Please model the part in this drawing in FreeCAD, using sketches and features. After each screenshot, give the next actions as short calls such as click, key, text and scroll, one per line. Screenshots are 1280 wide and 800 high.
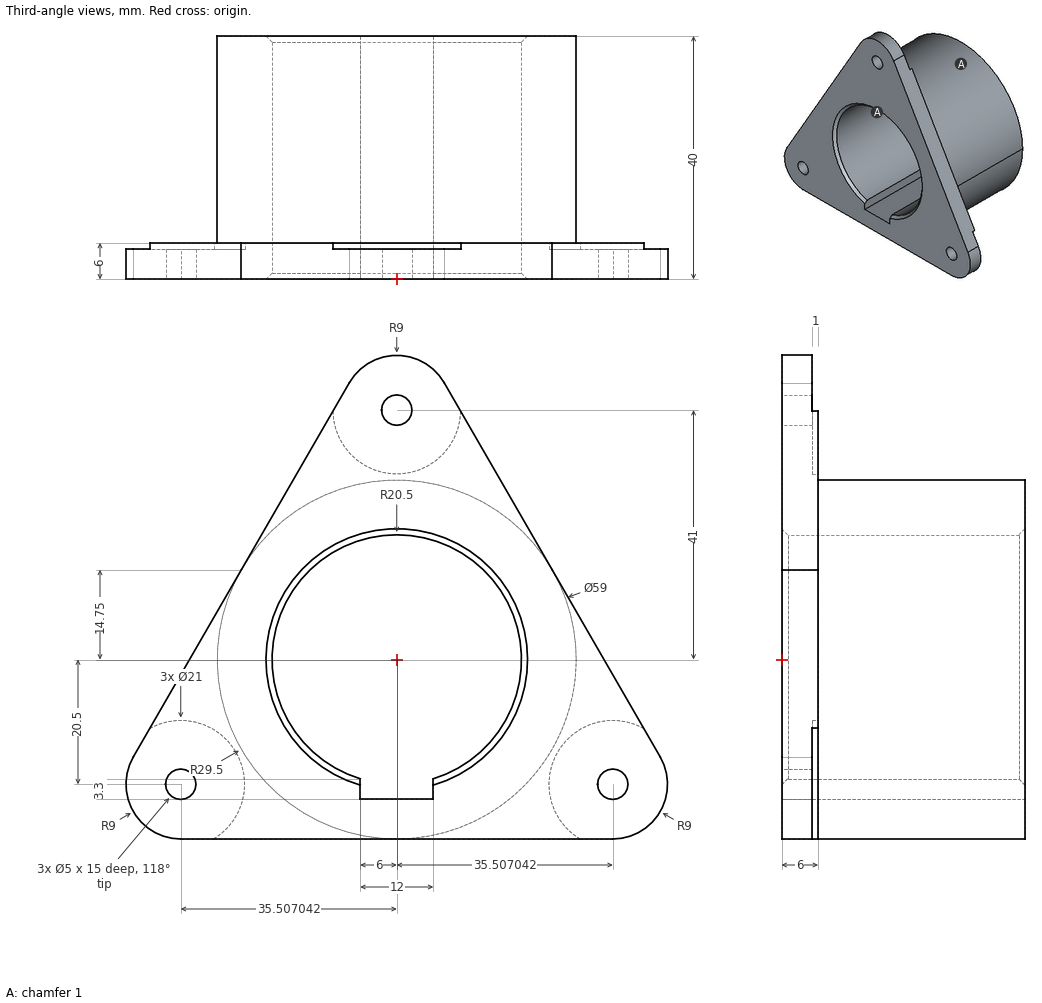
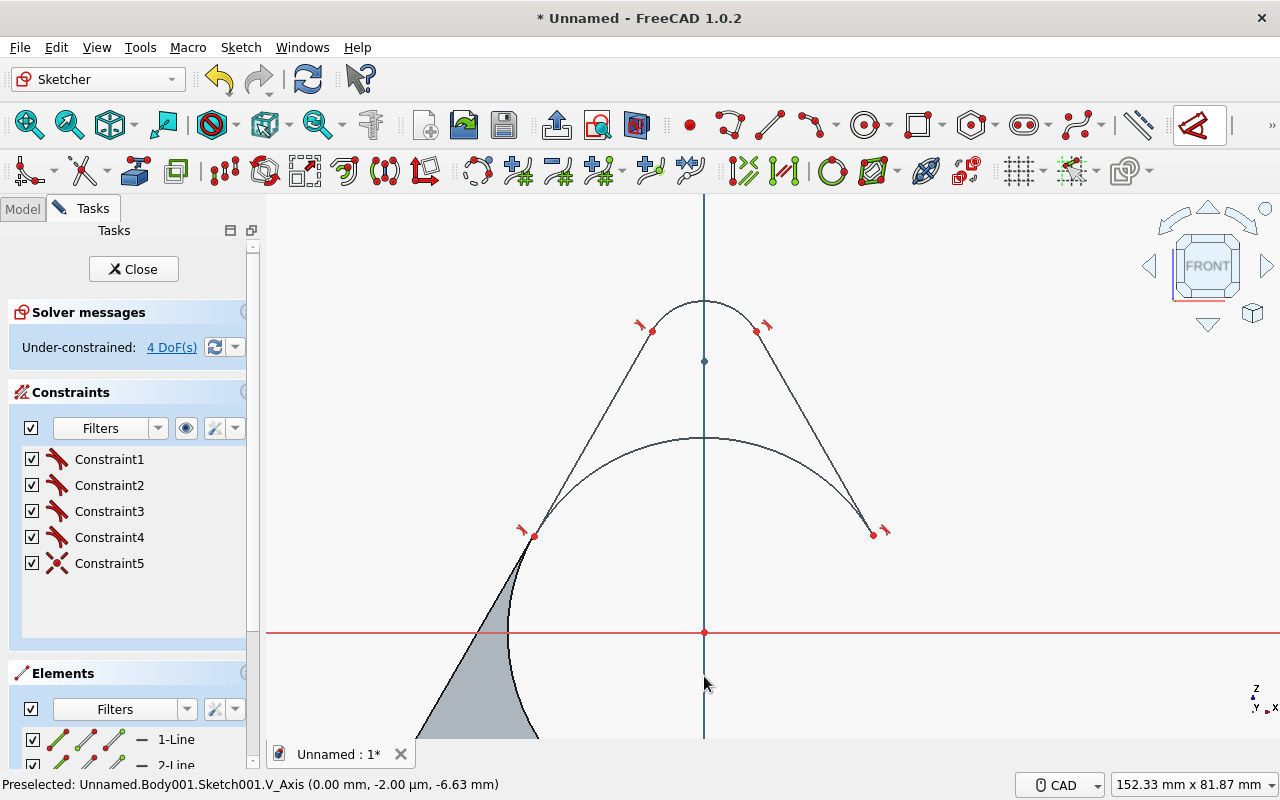
key(c)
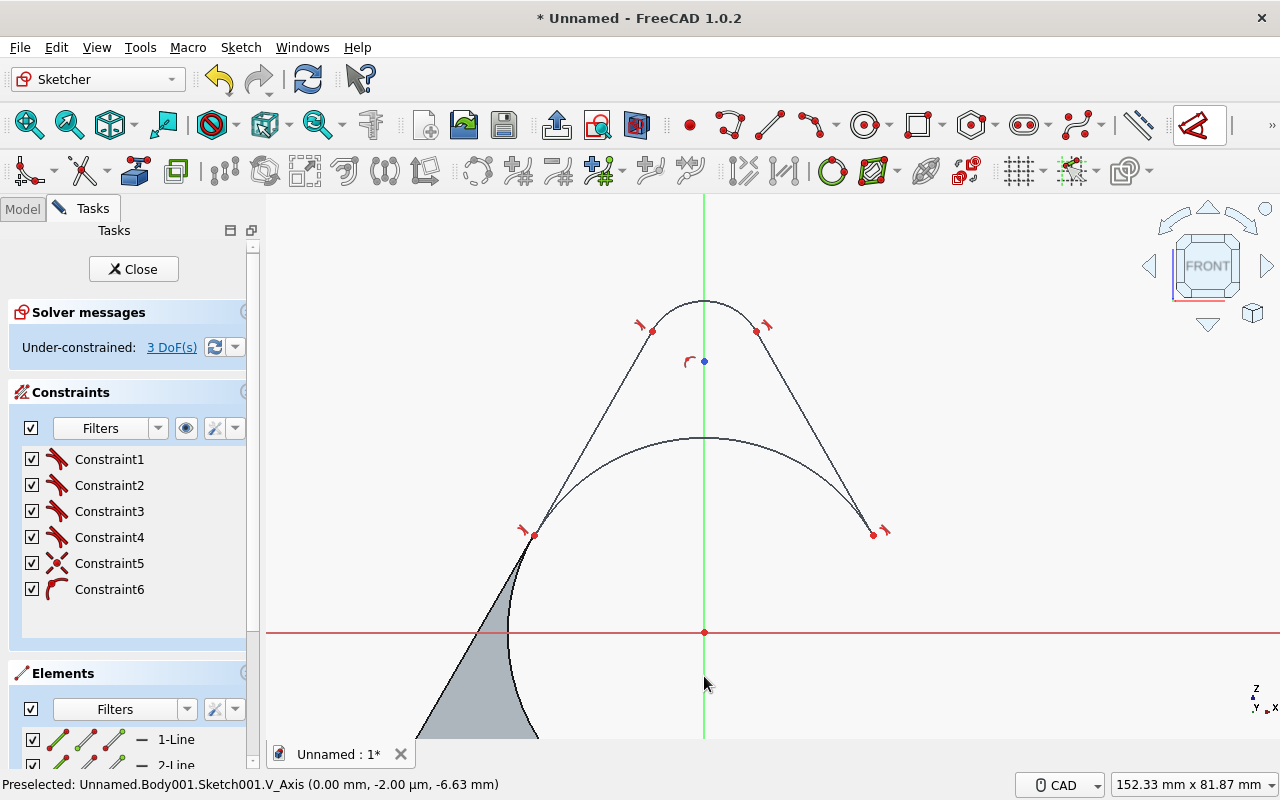
click(728, 306)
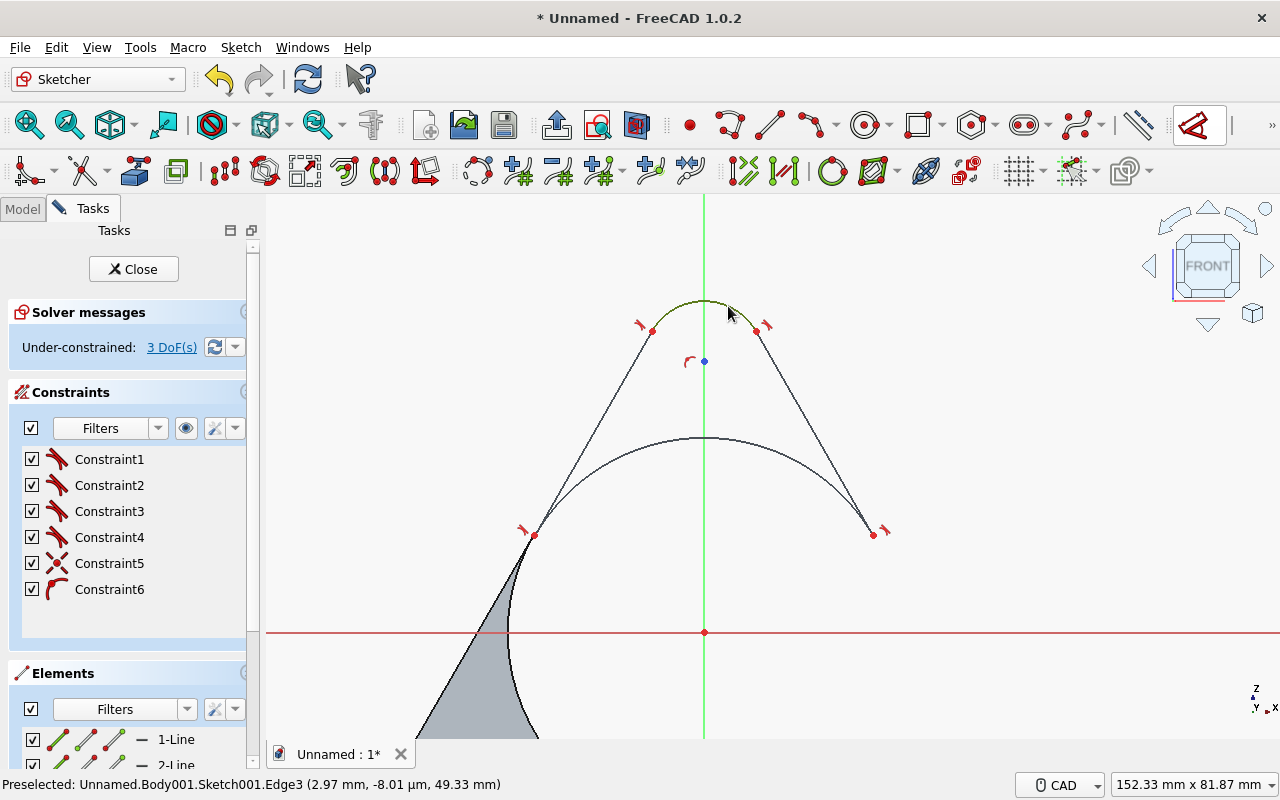
click(1220, 126)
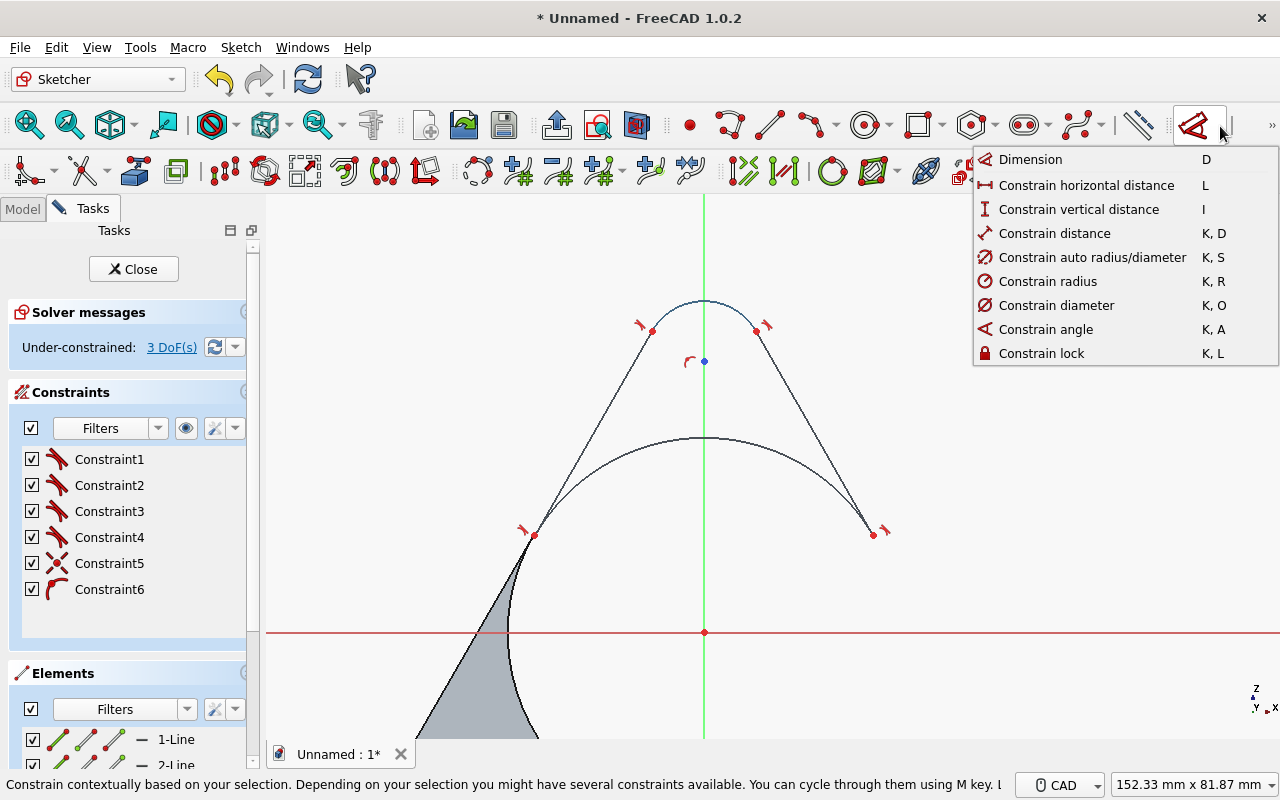
click(1126, 281)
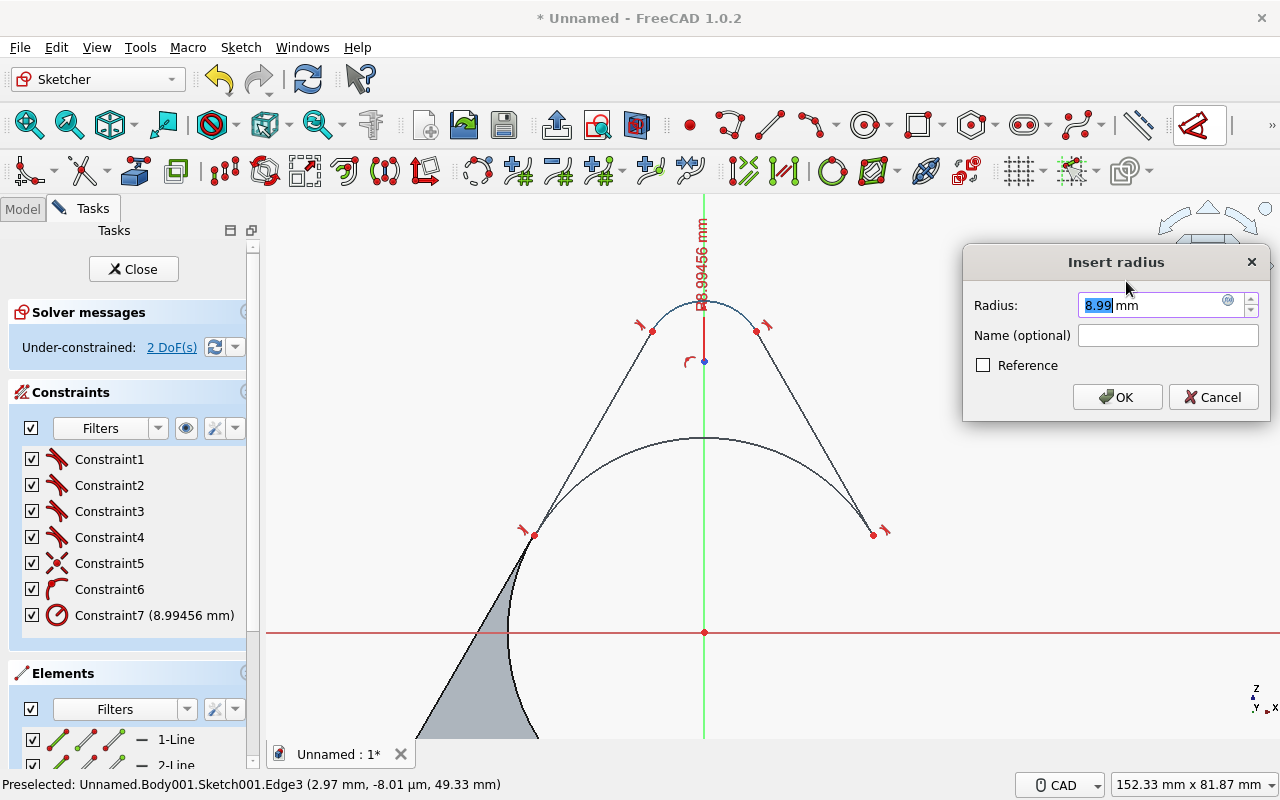
text(9)
key(Return)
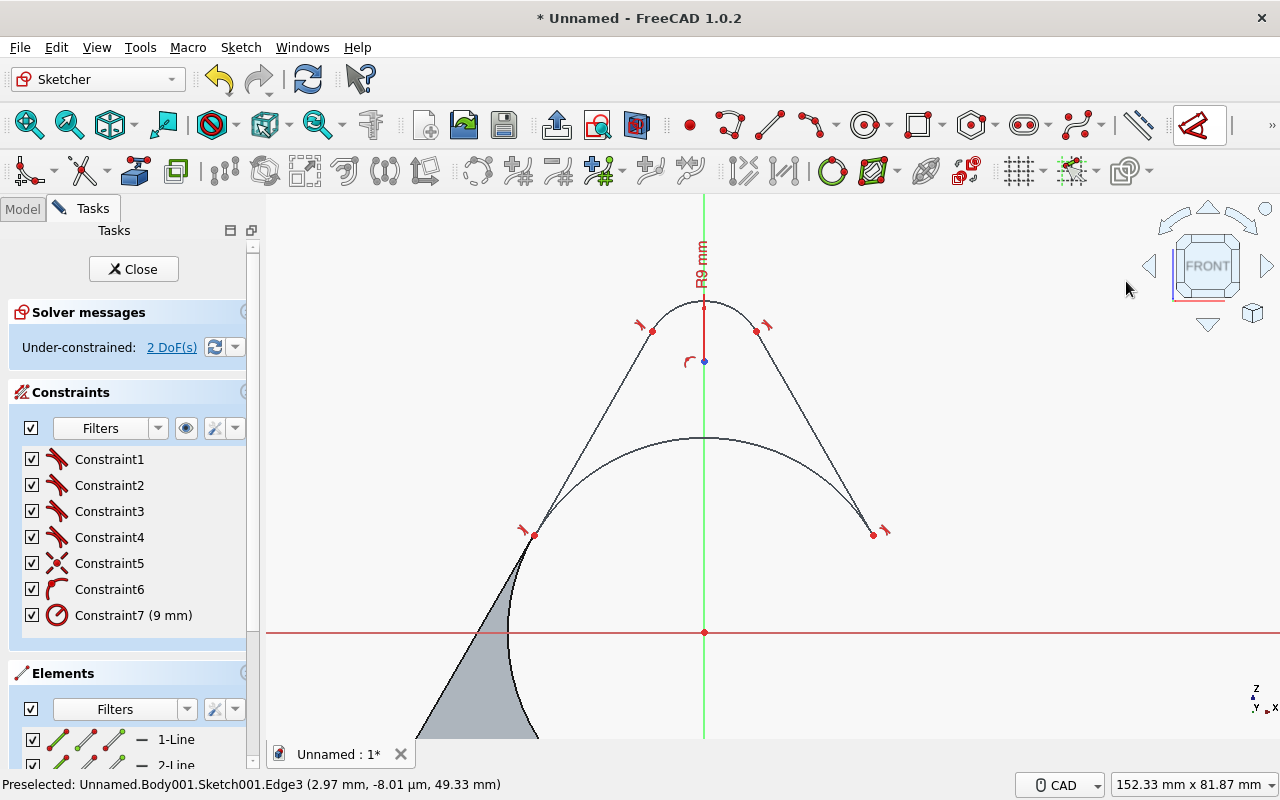
click(784, 455)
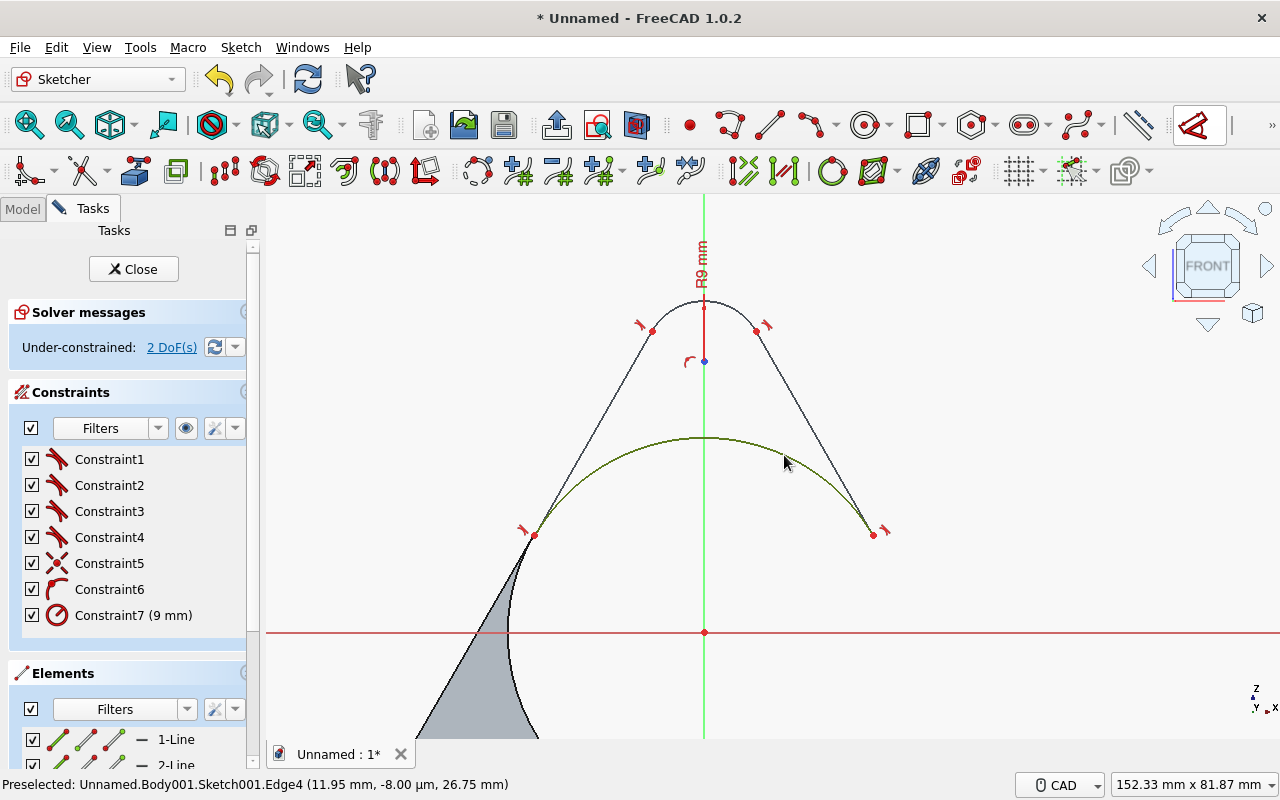
click(1220, 126)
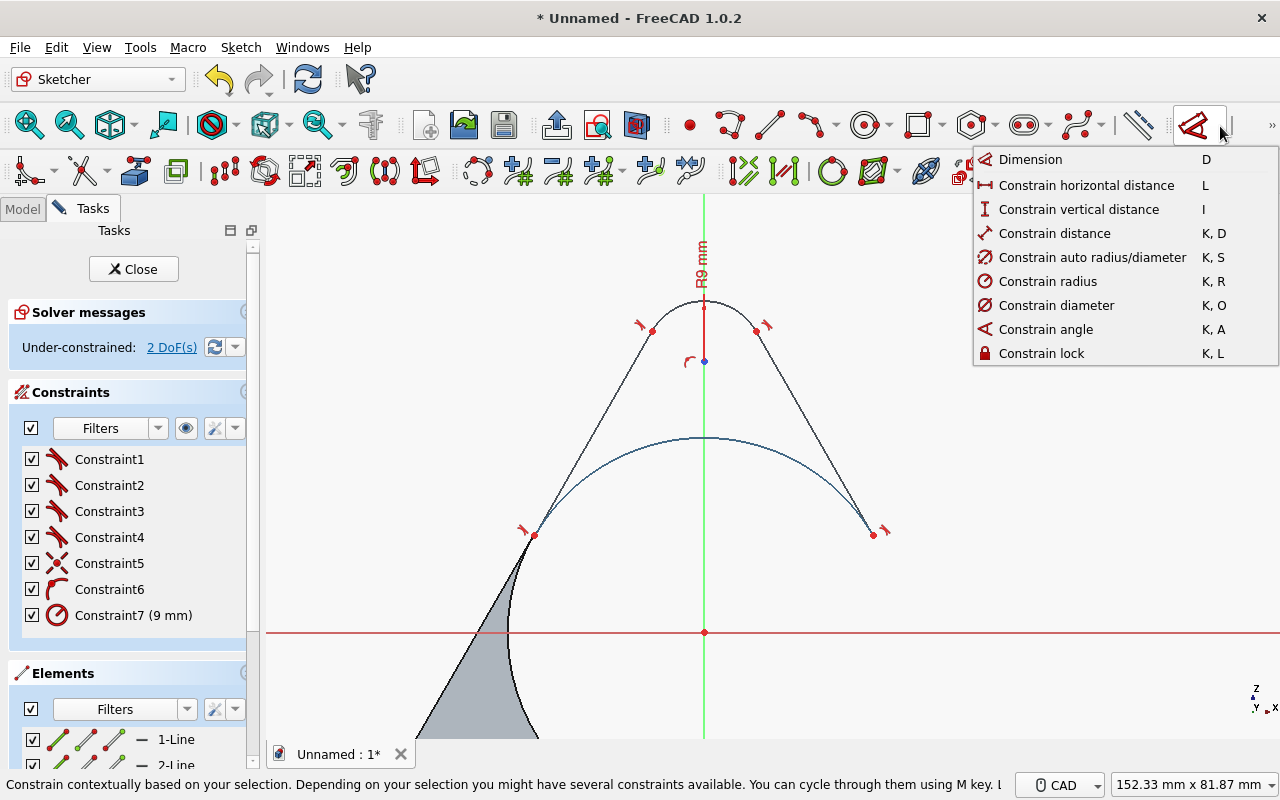
click(1126, 281)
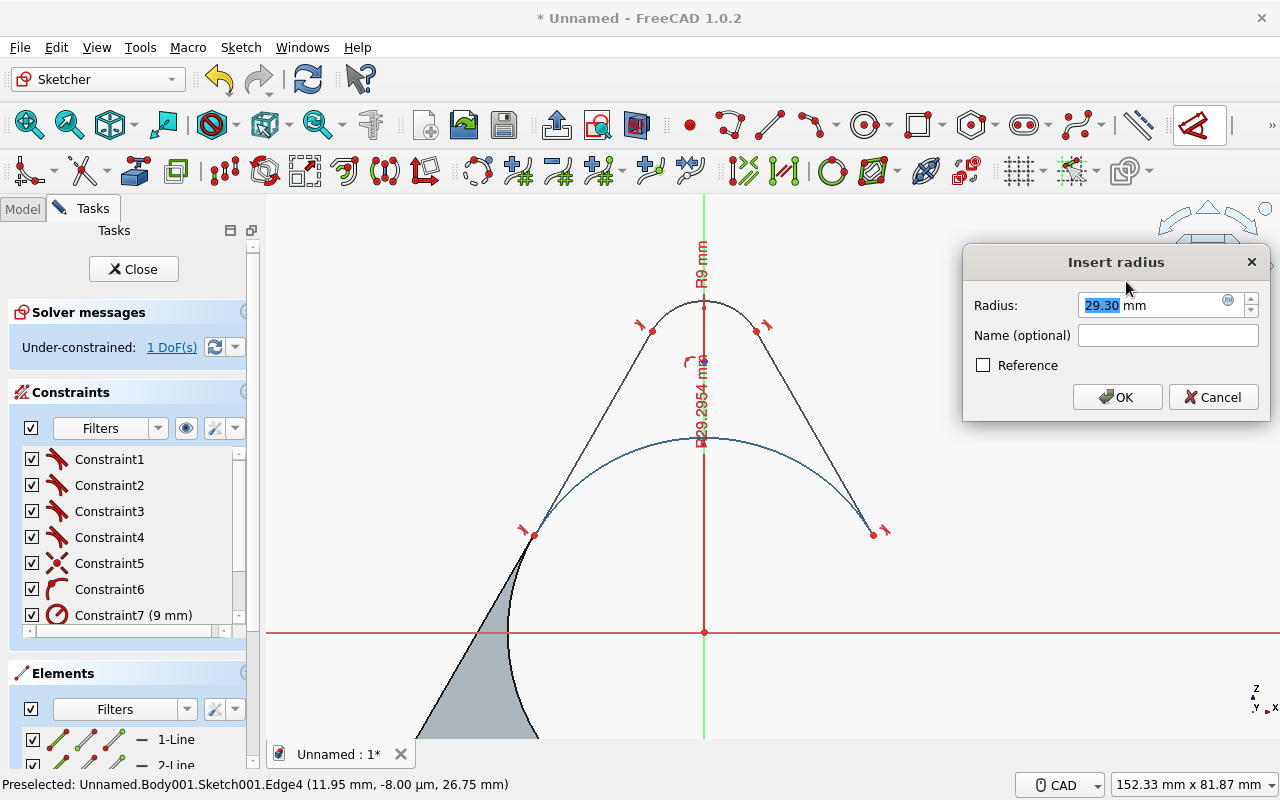
text(29.5)
key(Return)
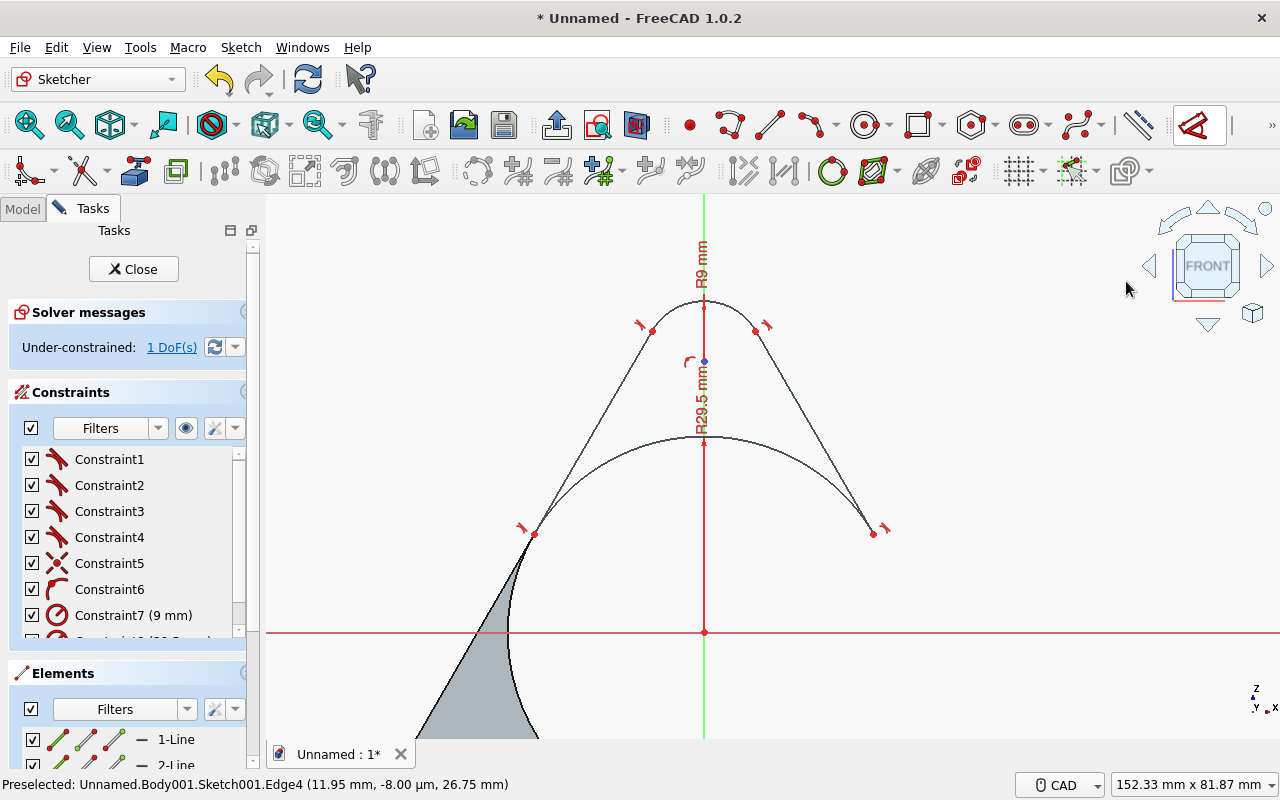
click(704, 361)